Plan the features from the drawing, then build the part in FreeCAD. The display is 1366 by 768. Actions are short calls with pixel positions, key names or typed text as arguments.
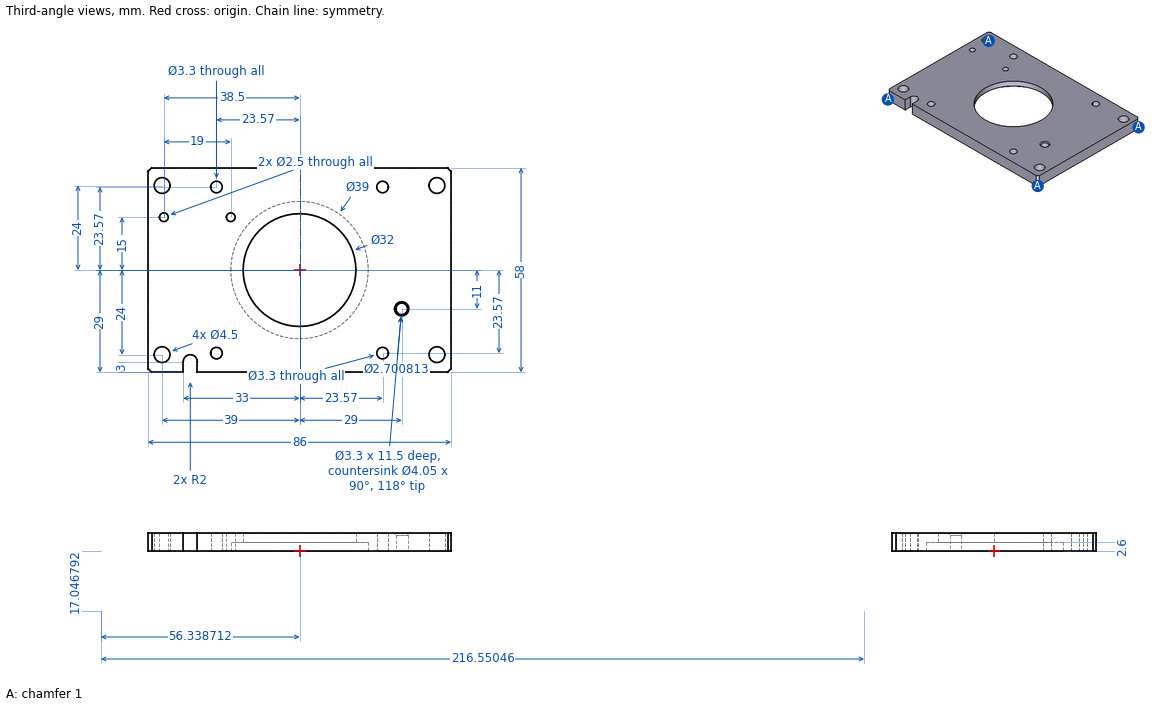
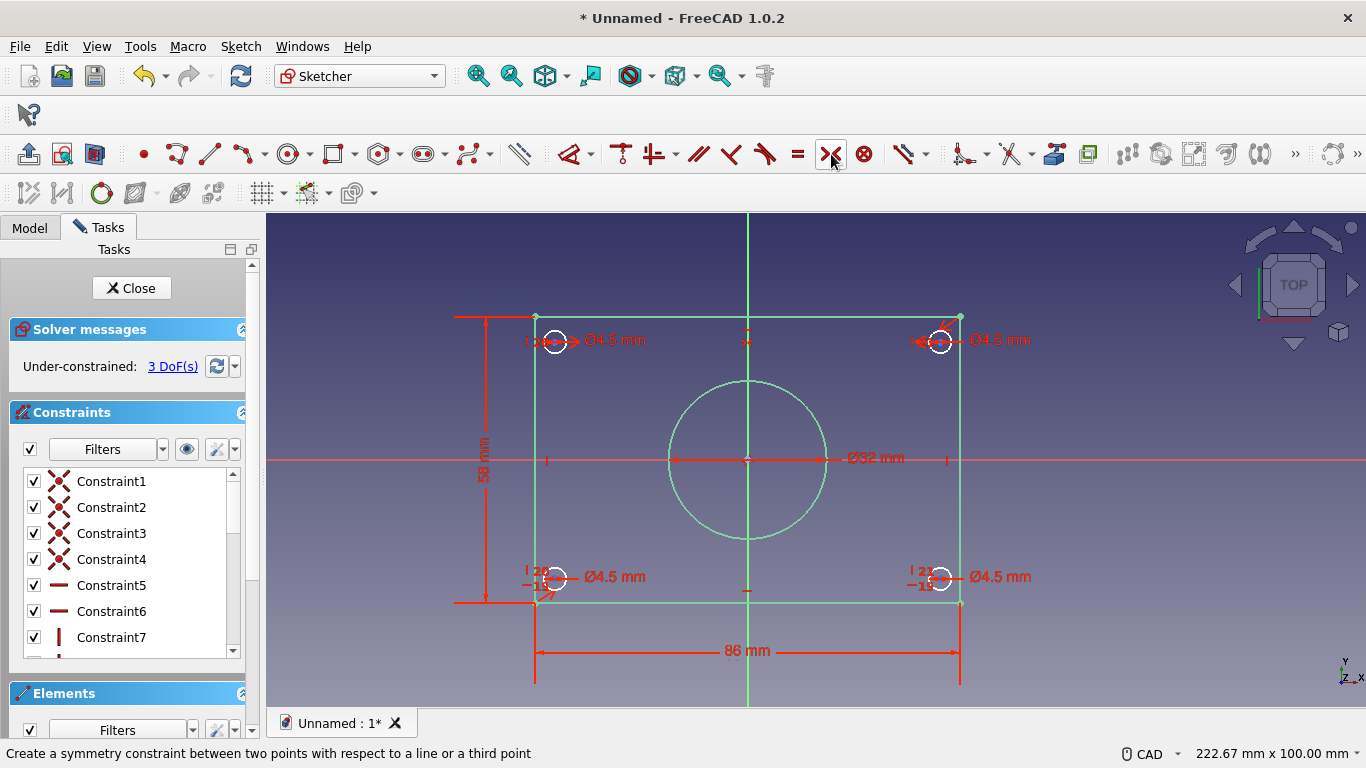
click(555, 579)
click(651, 426)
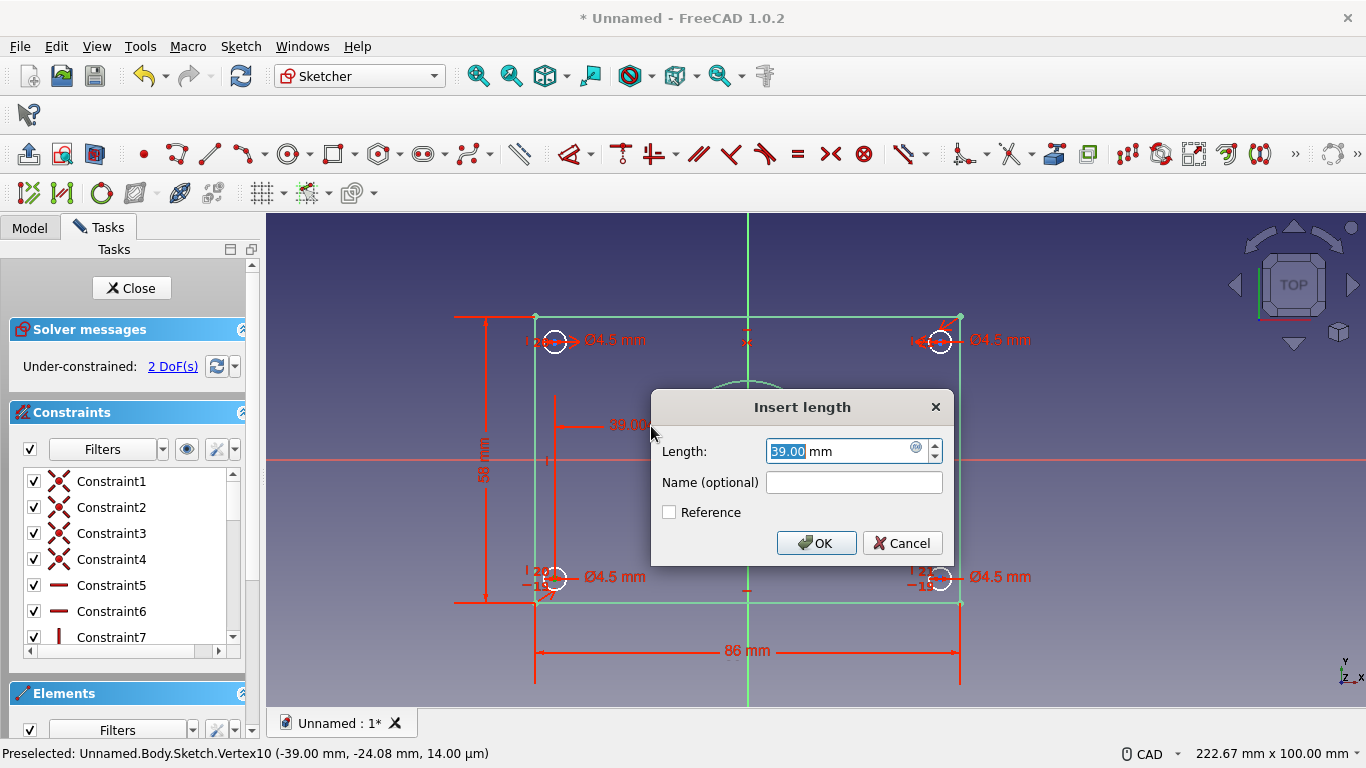
text(39)
key(Return)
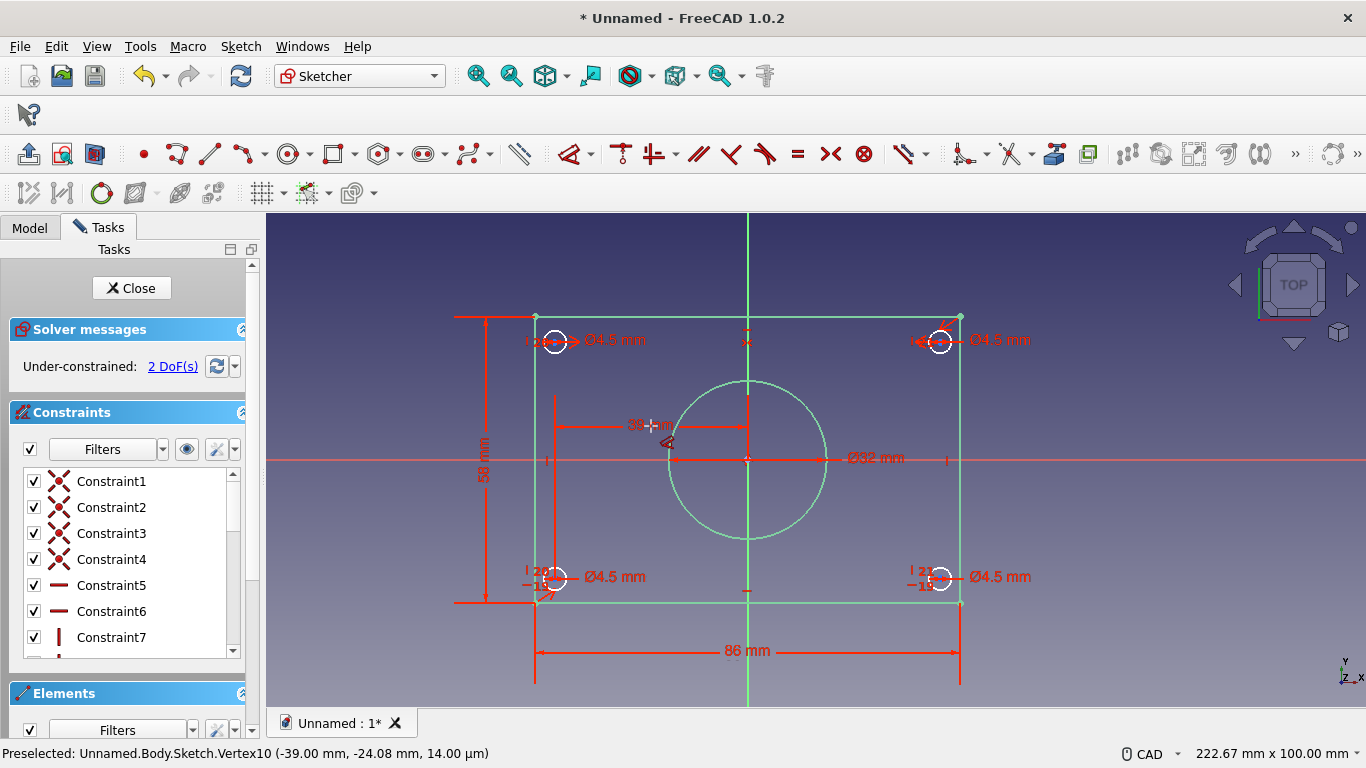
click(555, 579)
click(521, 519)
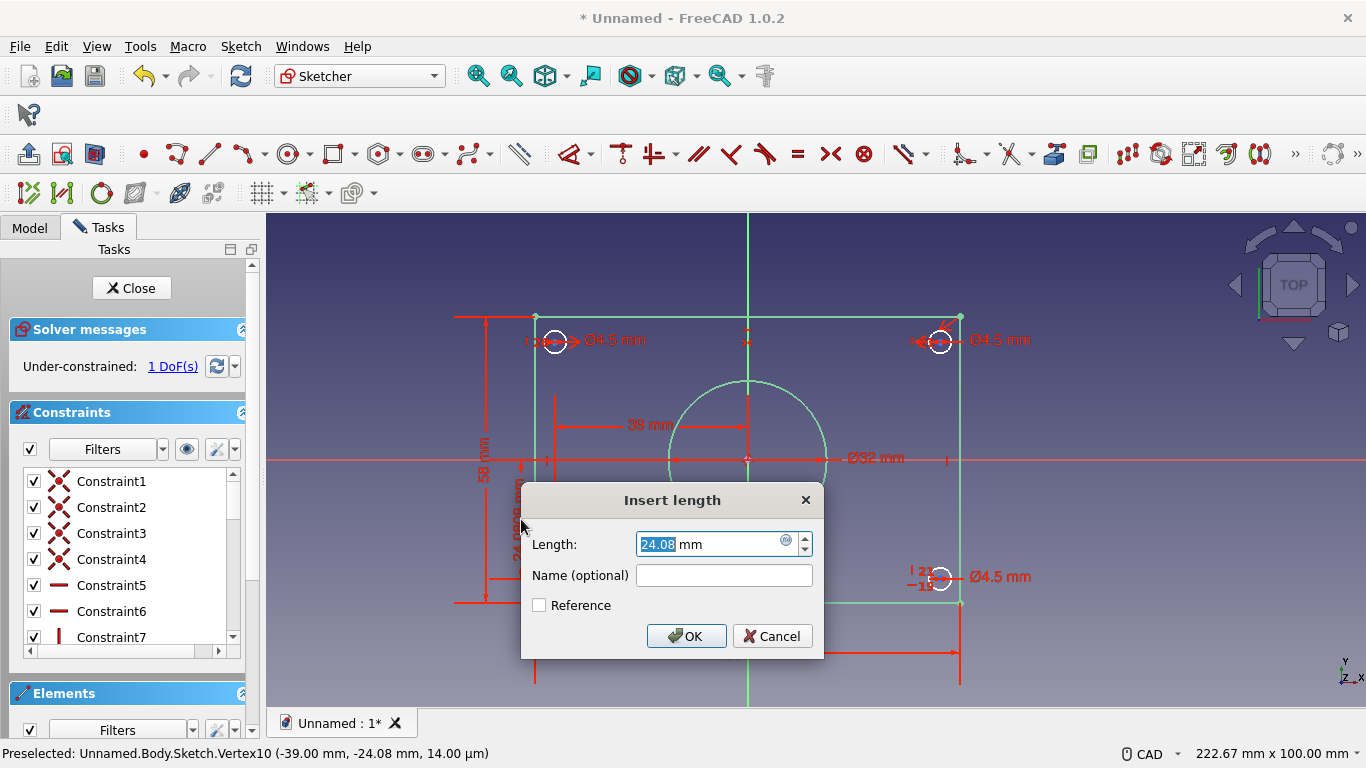
text(24)
key(Return)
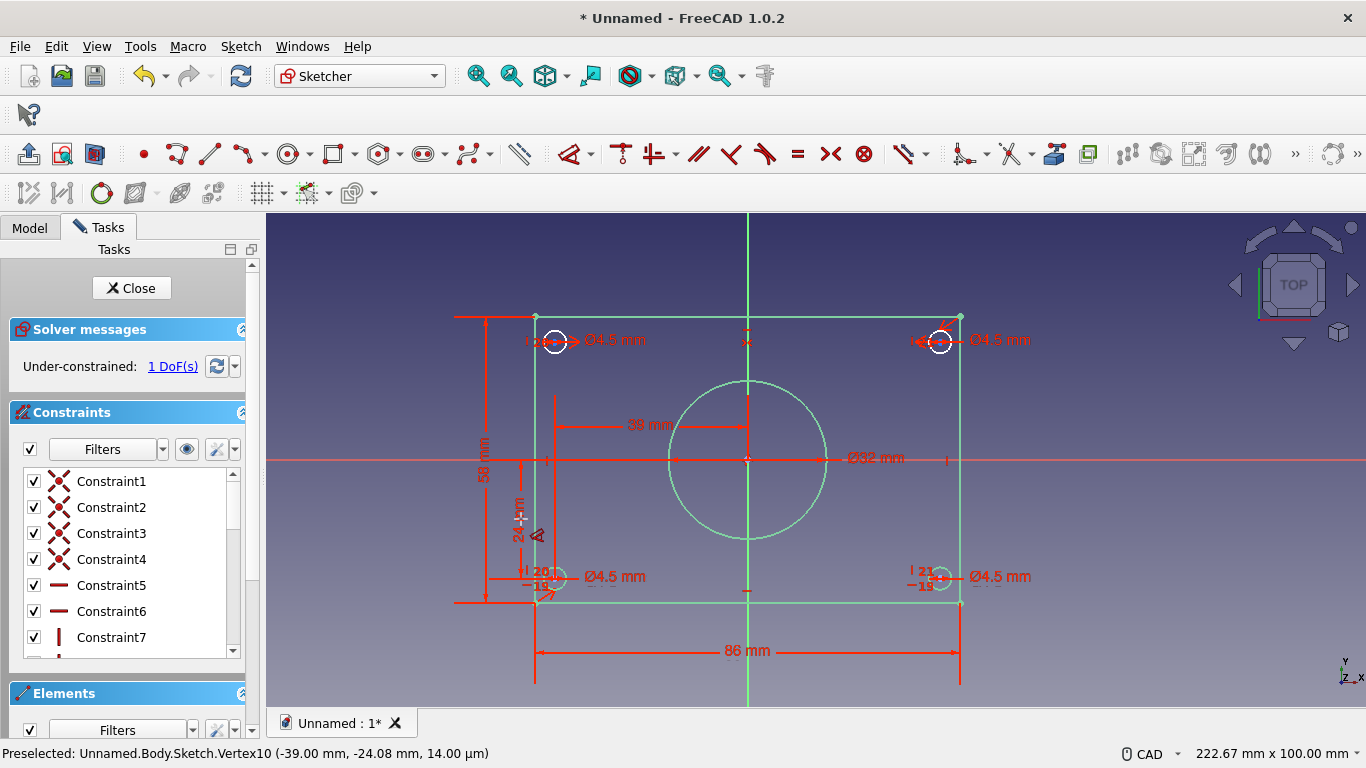
click(555, 342)
click(521, 401)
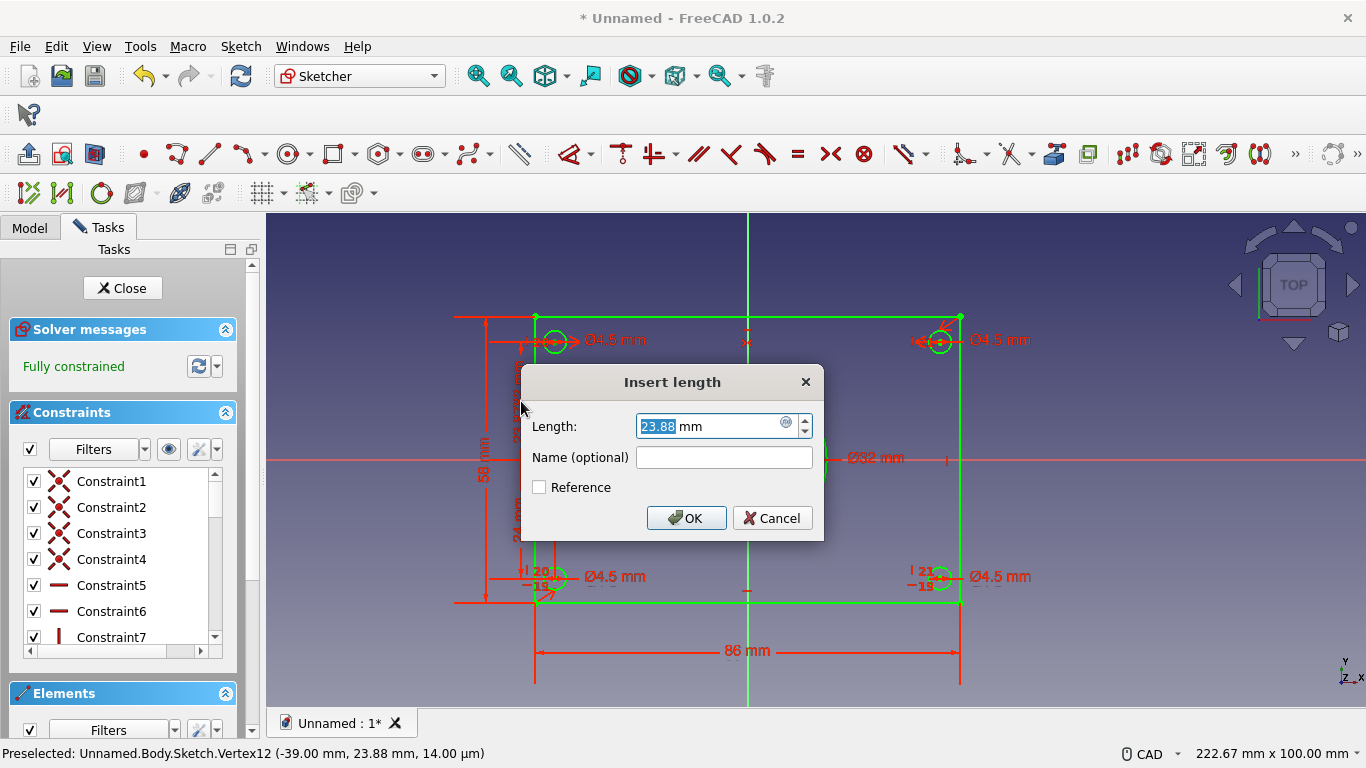
text(24)
key(Return)
key(Escape)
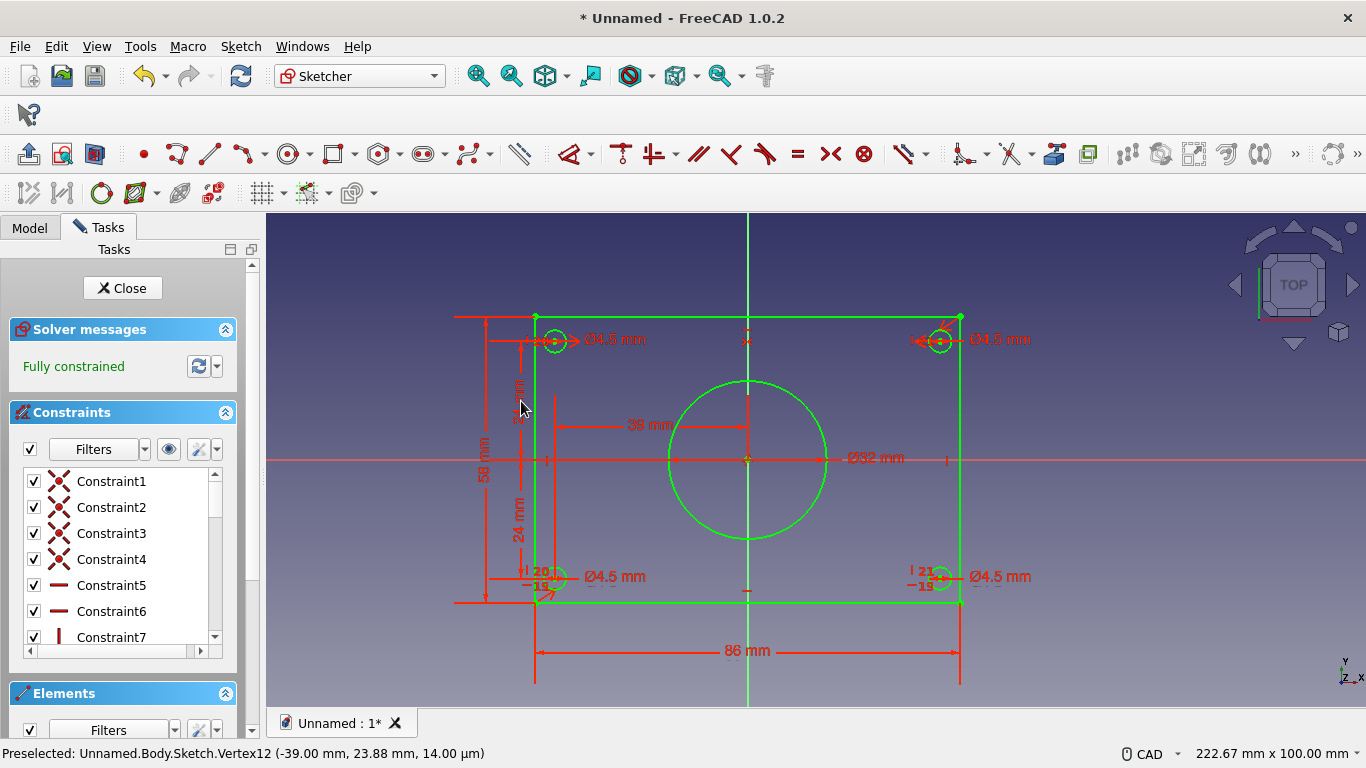
click(123, 288)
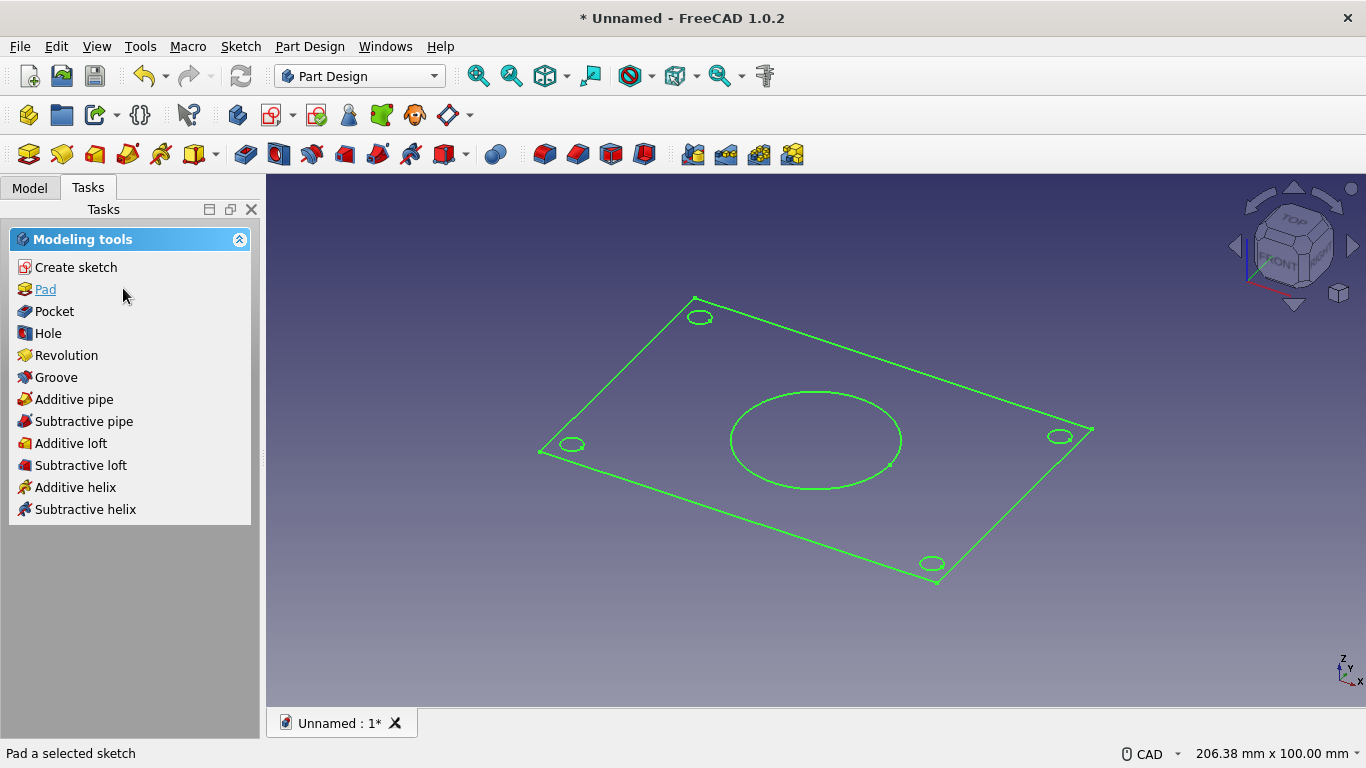
click(29, 154)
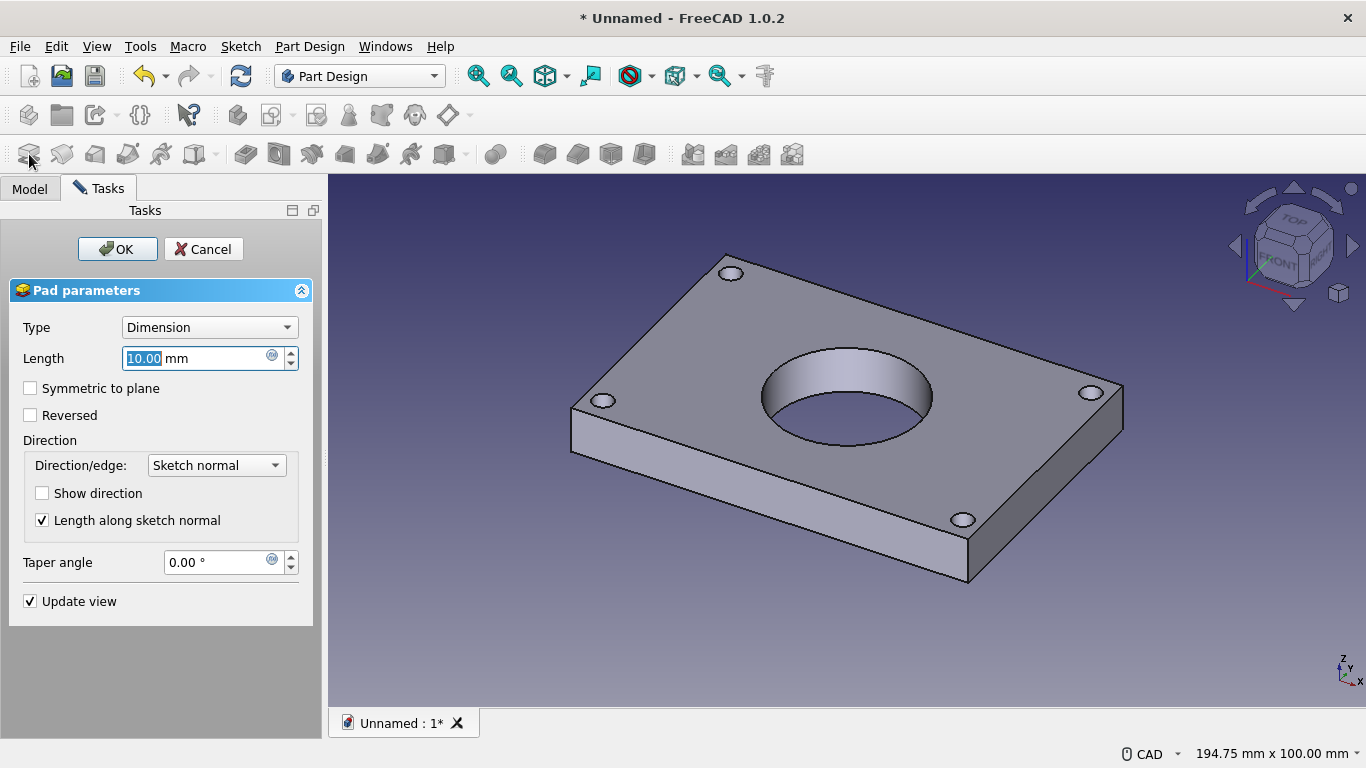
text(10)
key(Tab)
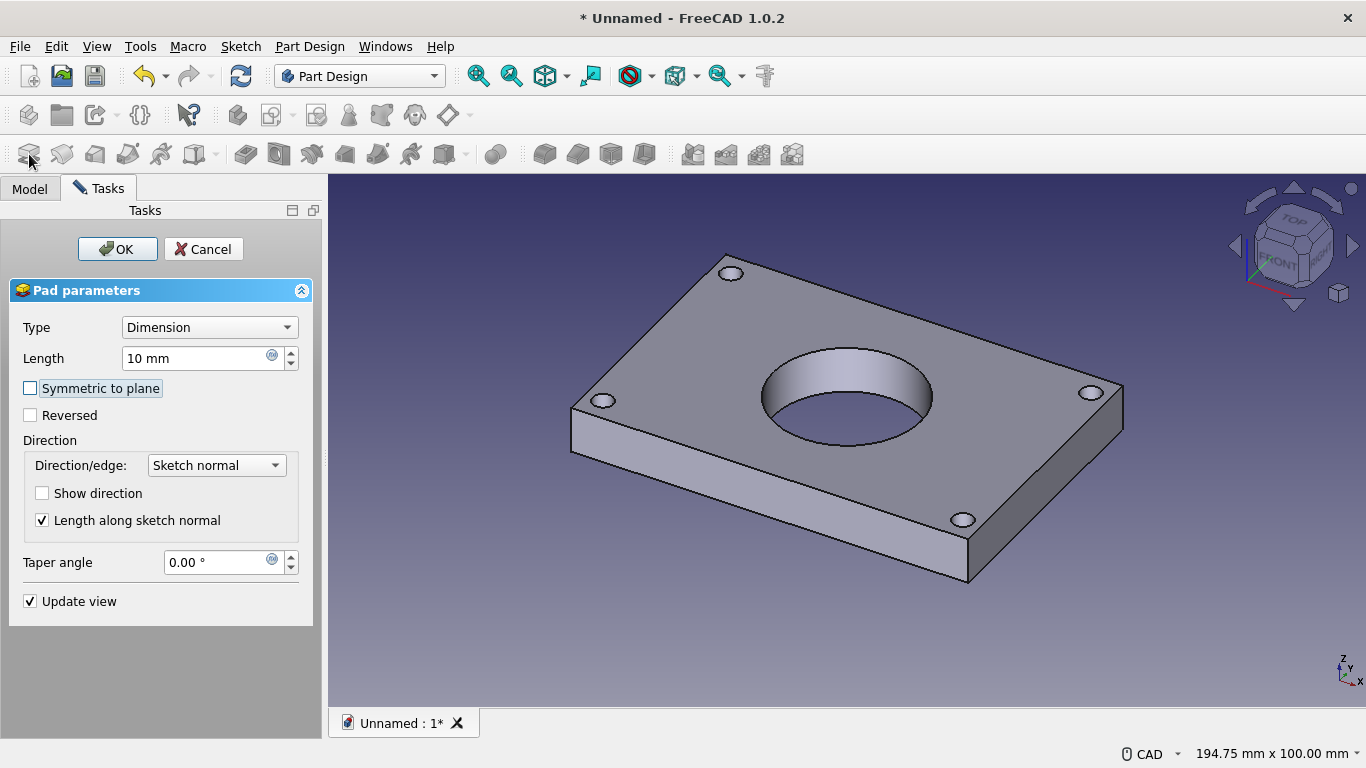
click(31, 388)